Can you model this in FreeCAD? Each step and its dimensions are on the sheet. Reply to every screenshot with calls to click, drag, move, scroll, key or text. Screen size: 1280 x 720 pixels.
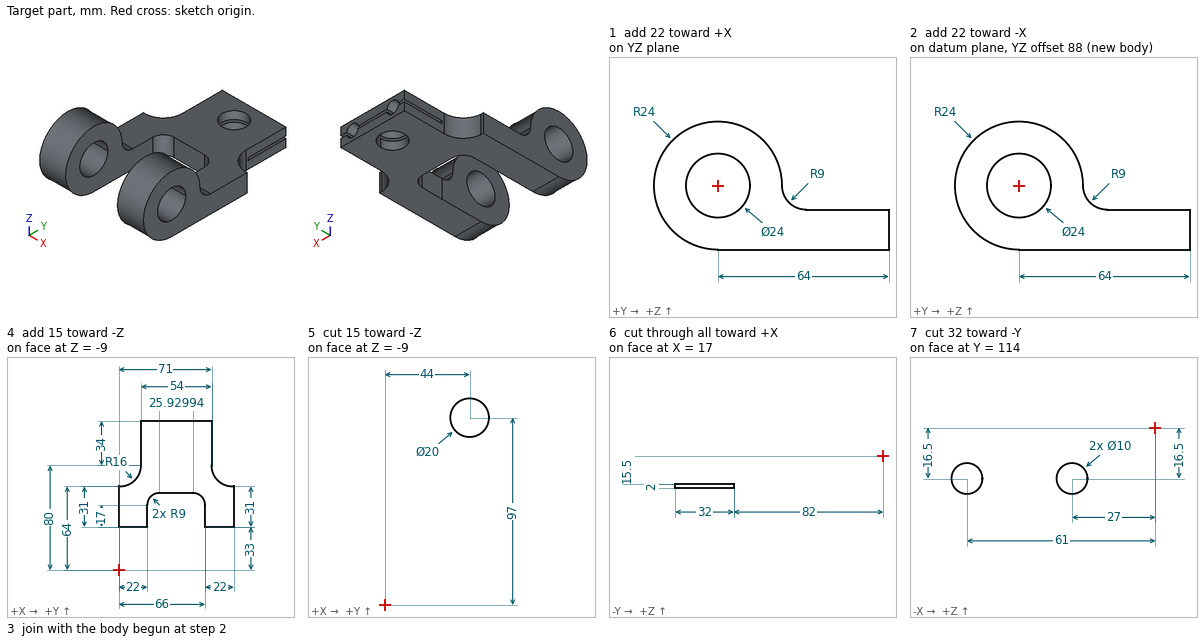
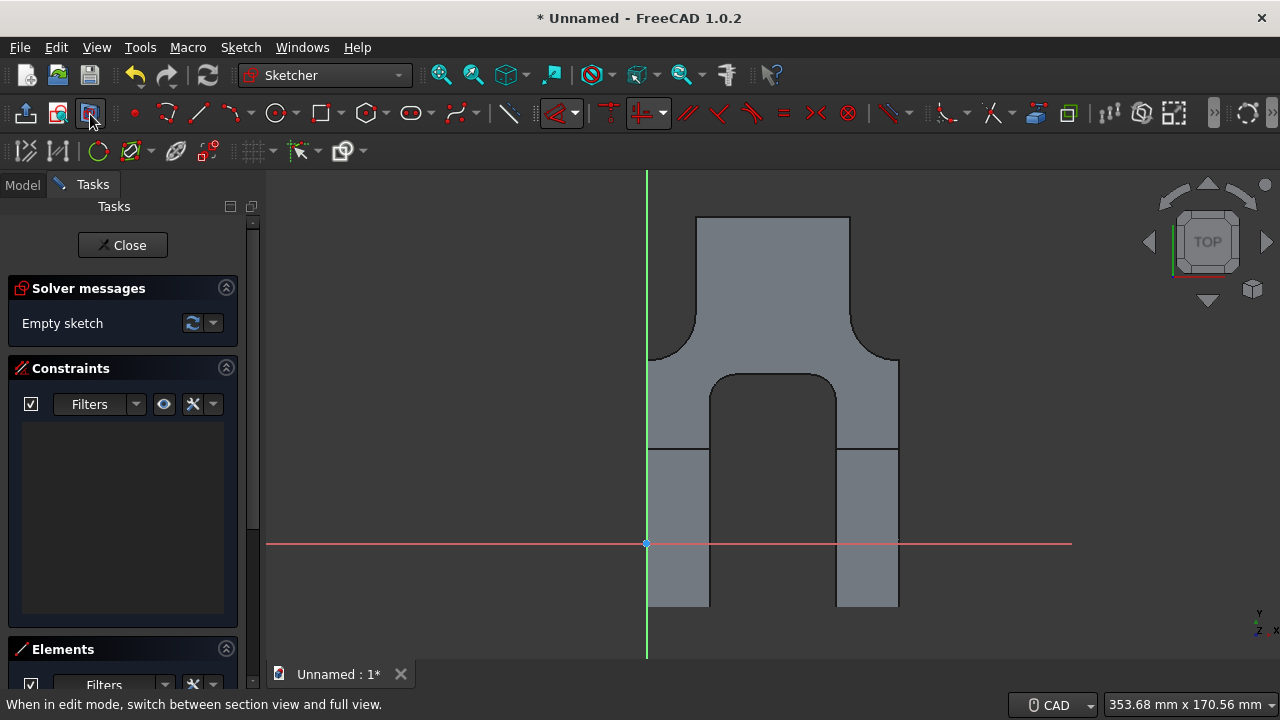
scroll(790, 228, up, 8)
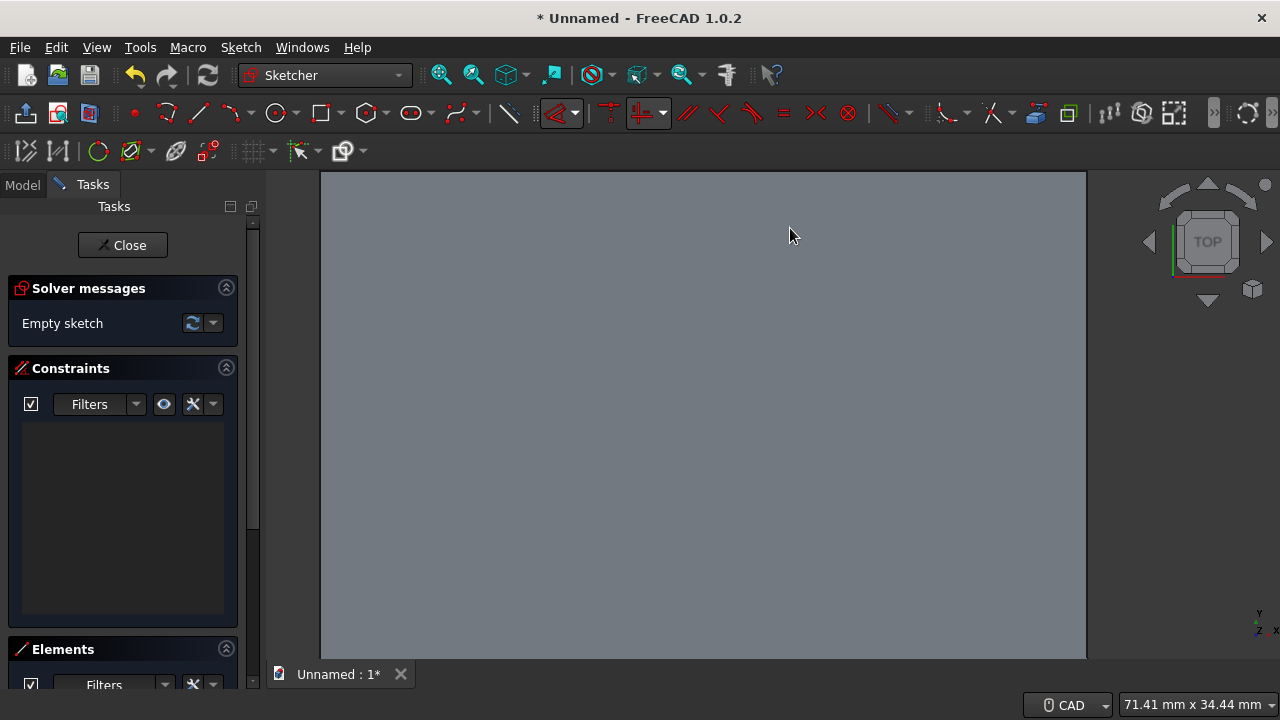
click(276, 114)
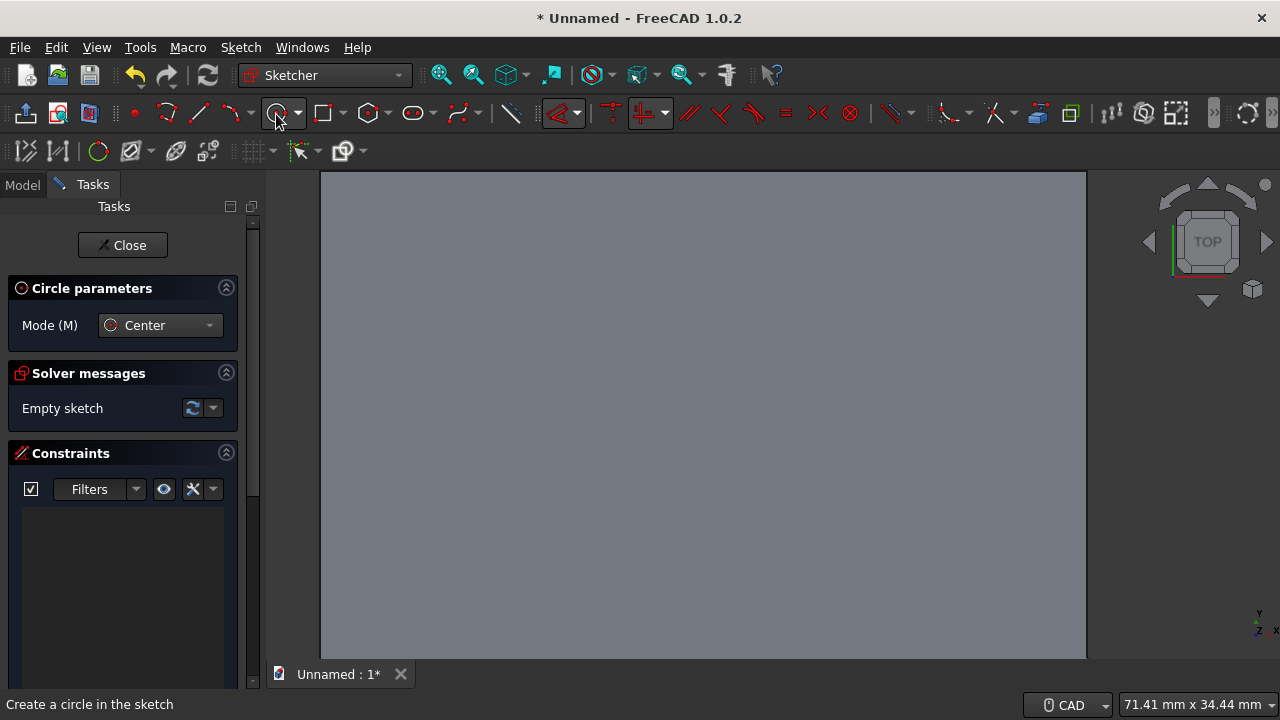
click(704, 413)
click(804, 312)
key(Escape)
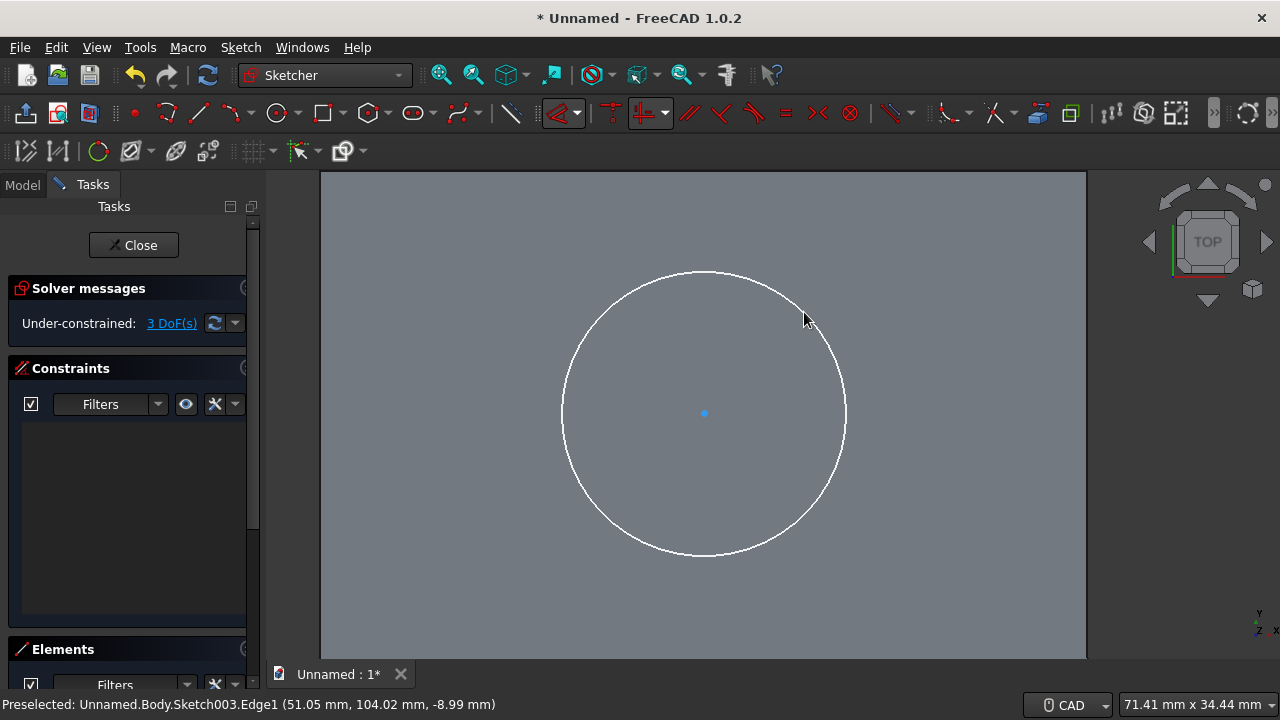
click(804, 313)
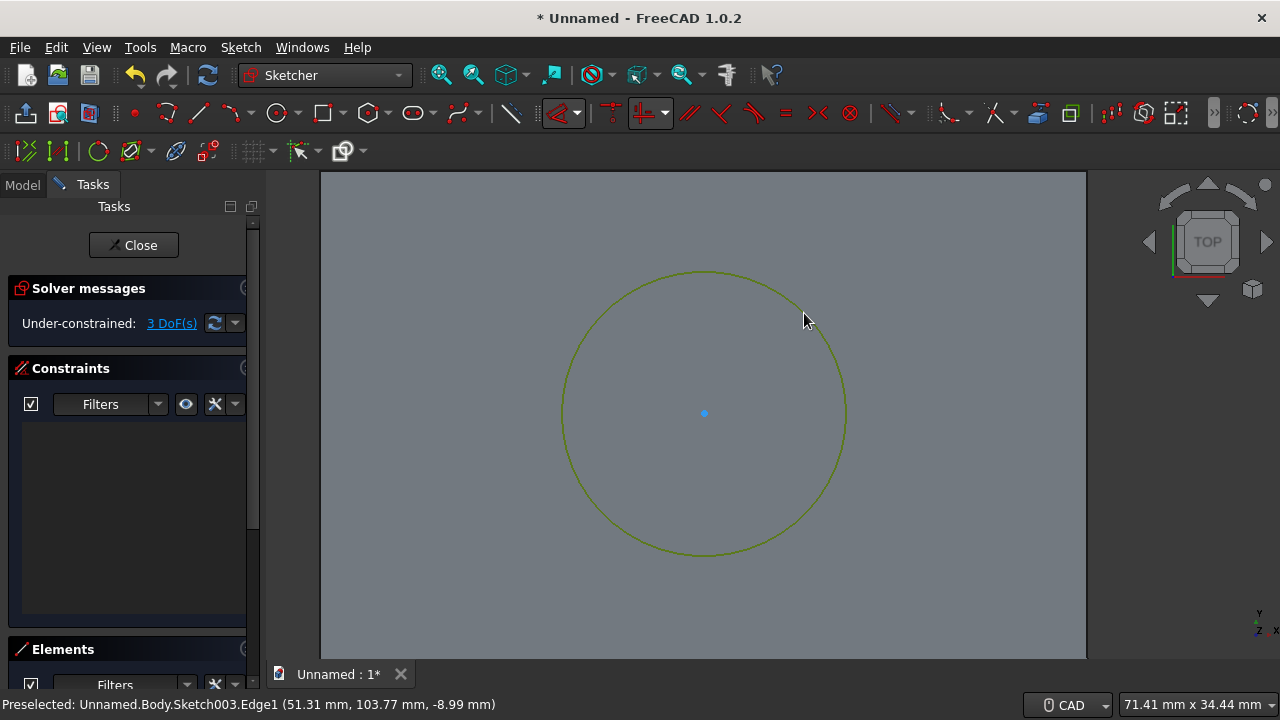
key(k)
key(o)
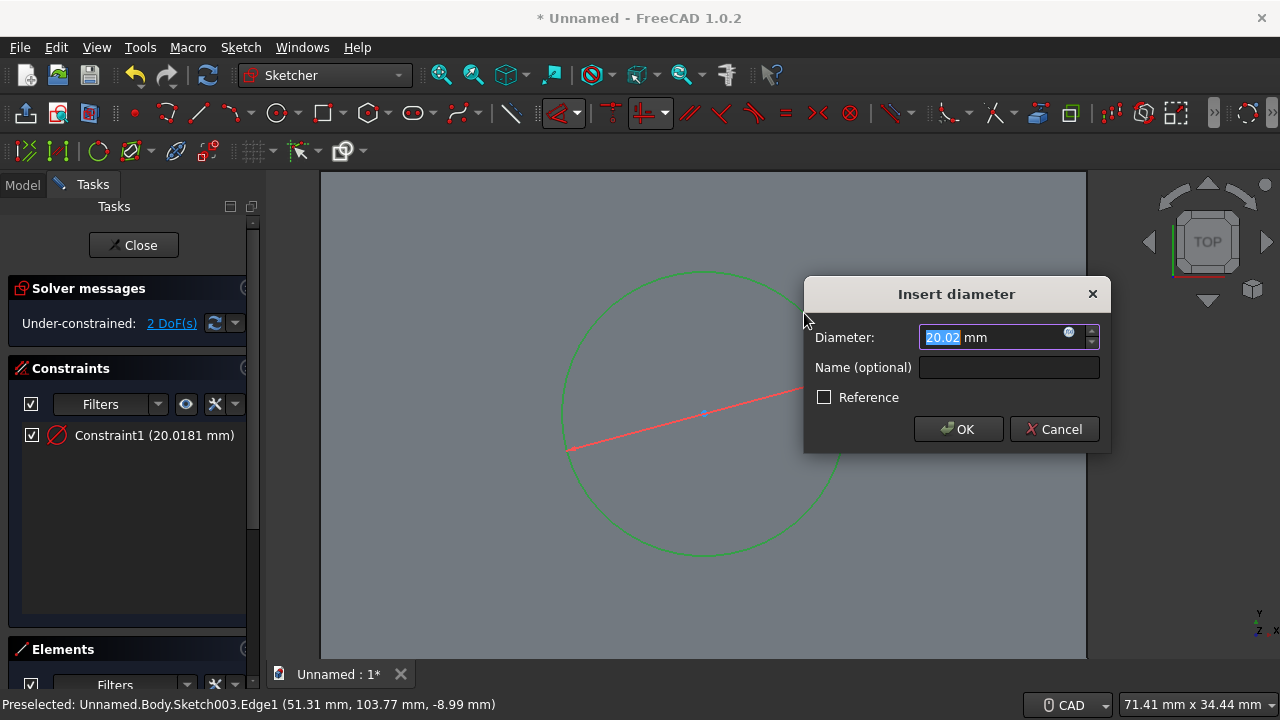
text(20)
key(Return)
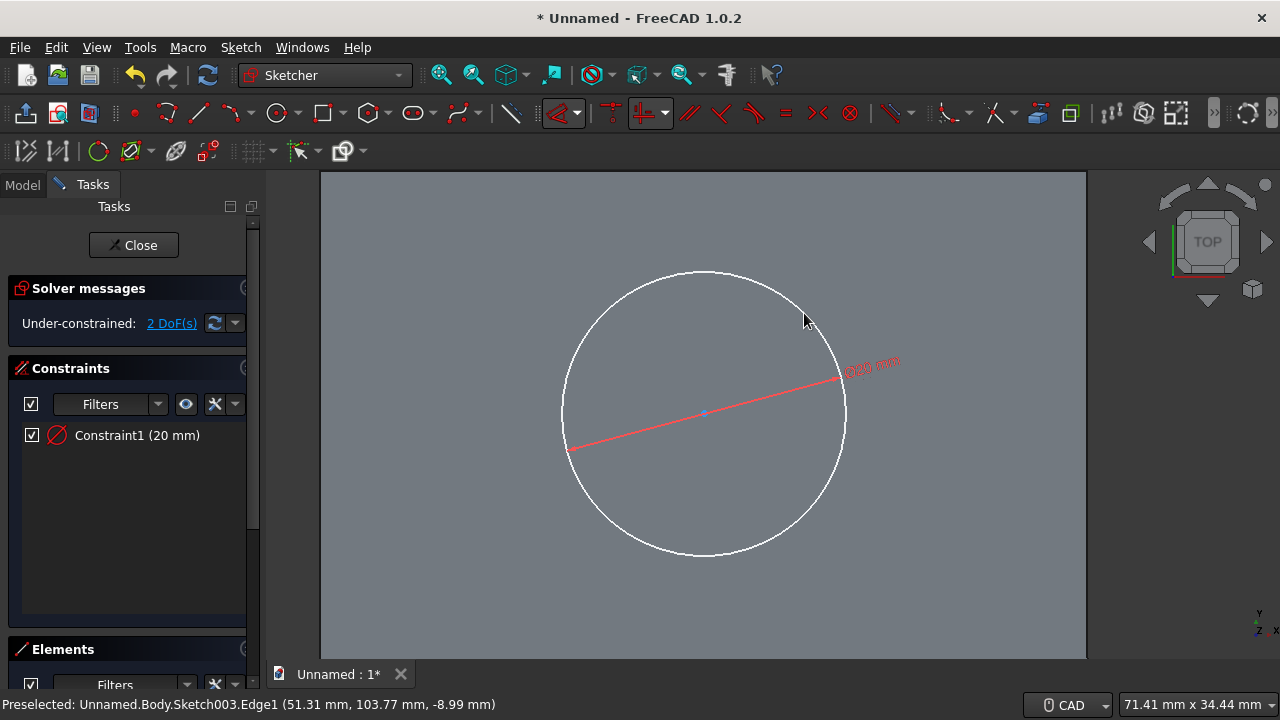
click(704, 414)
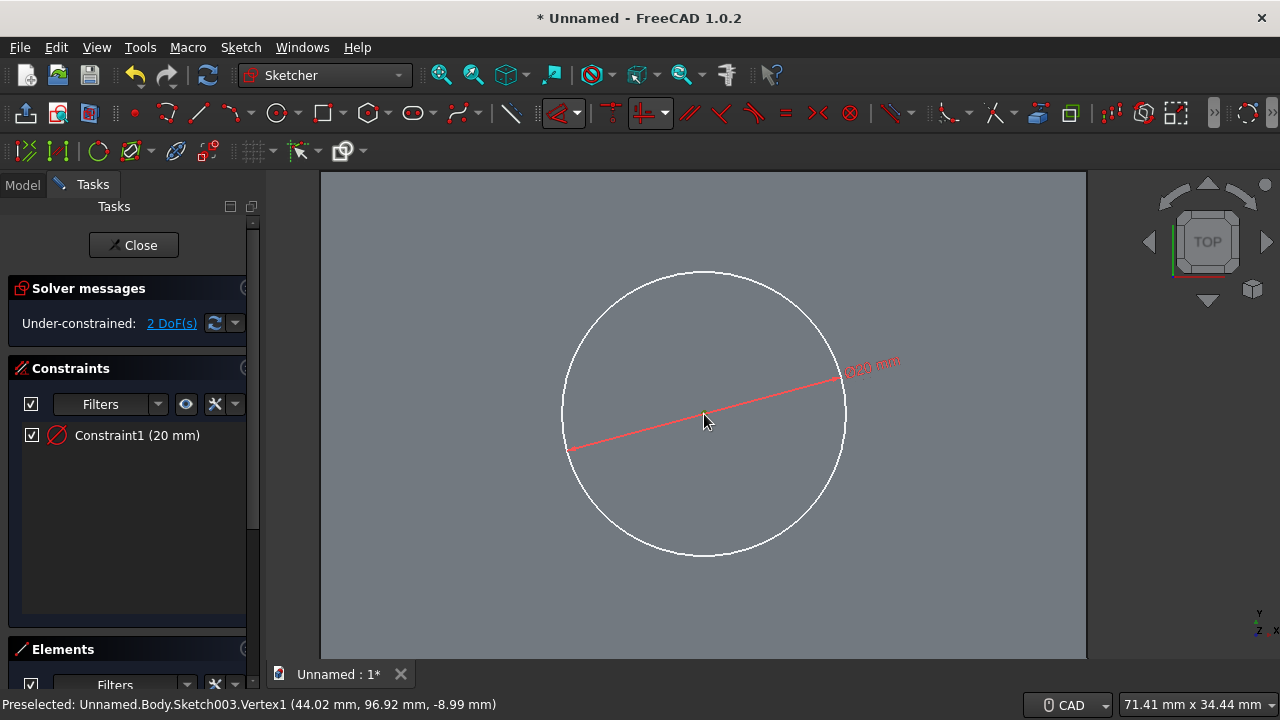
key(l)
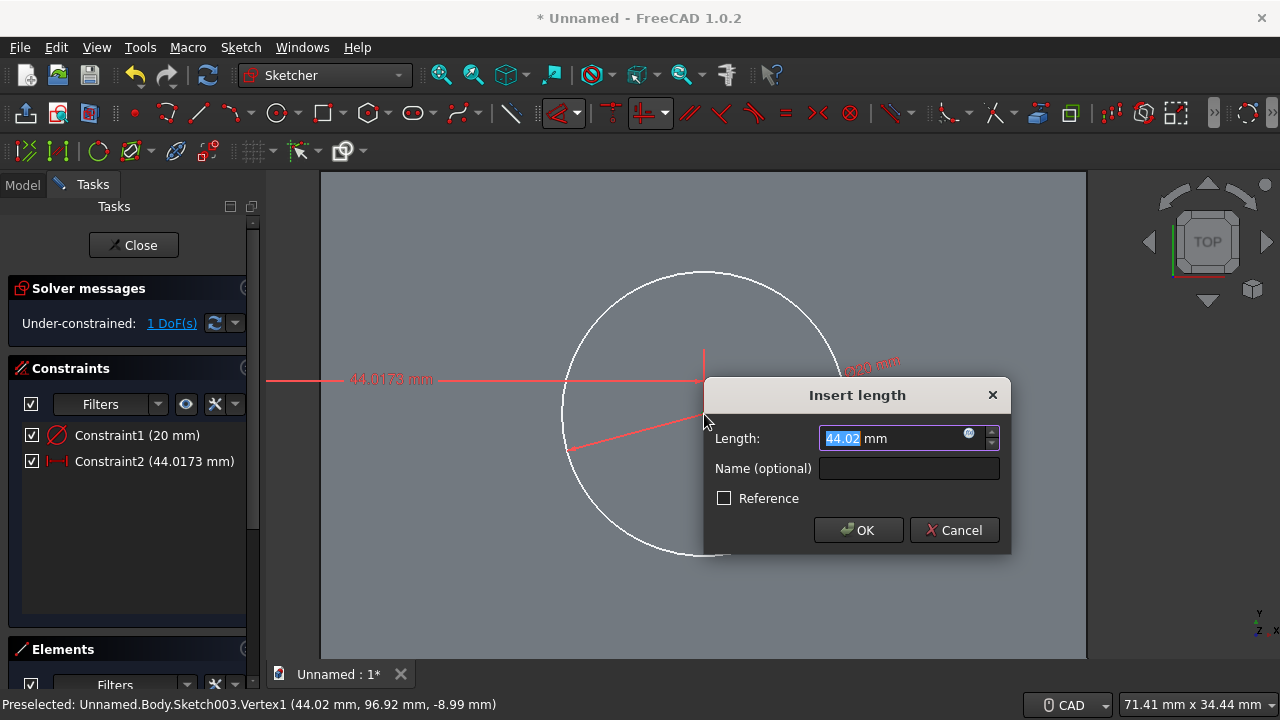
text(44)
key(Return)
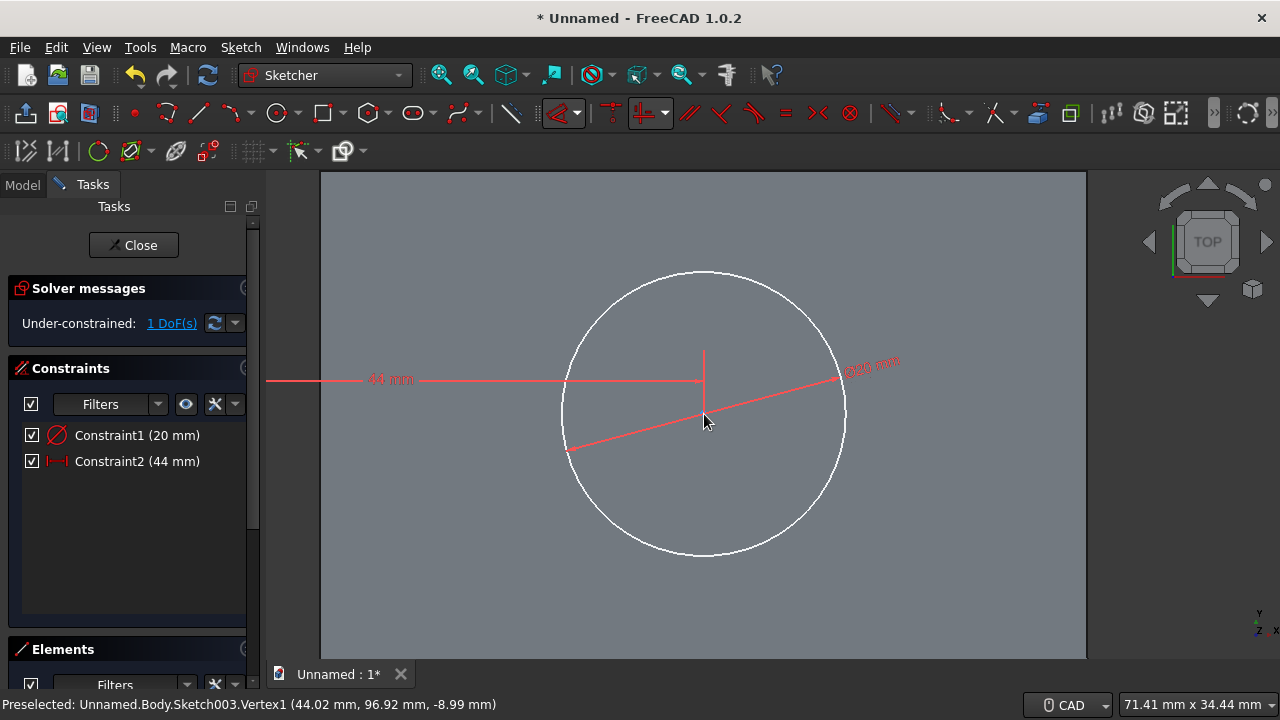
click(704, 414)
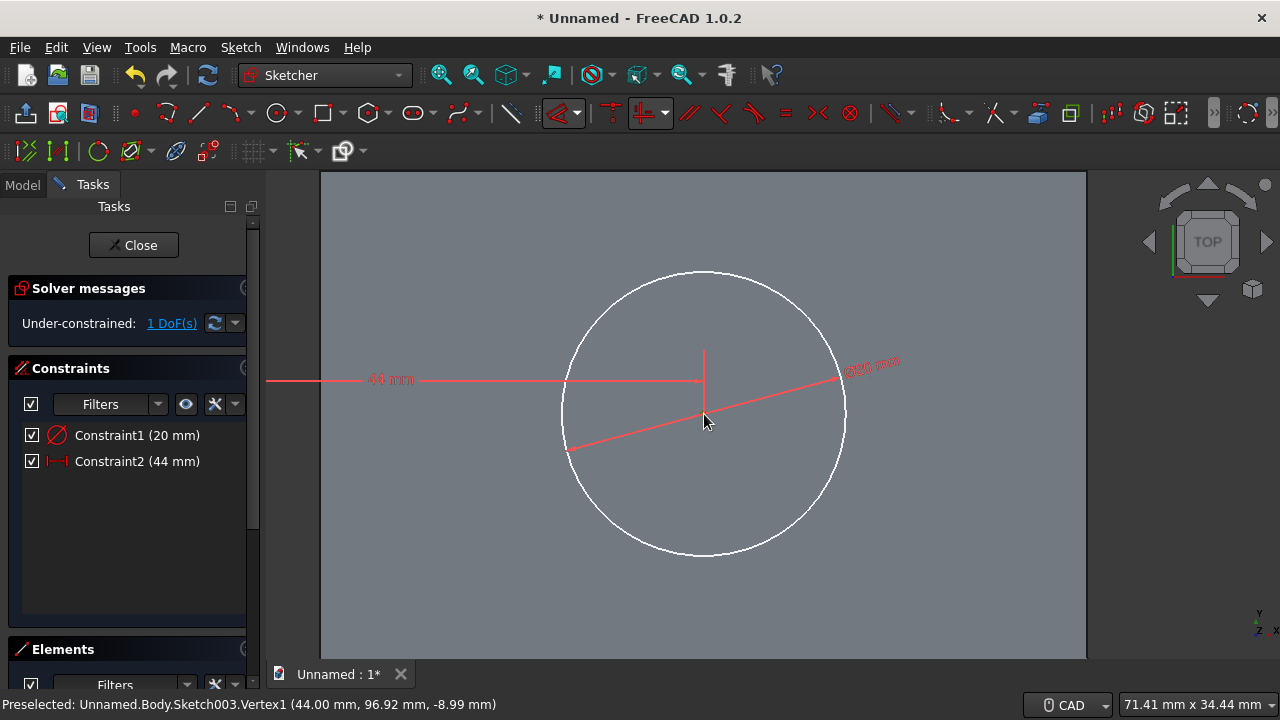
click(580, 114)